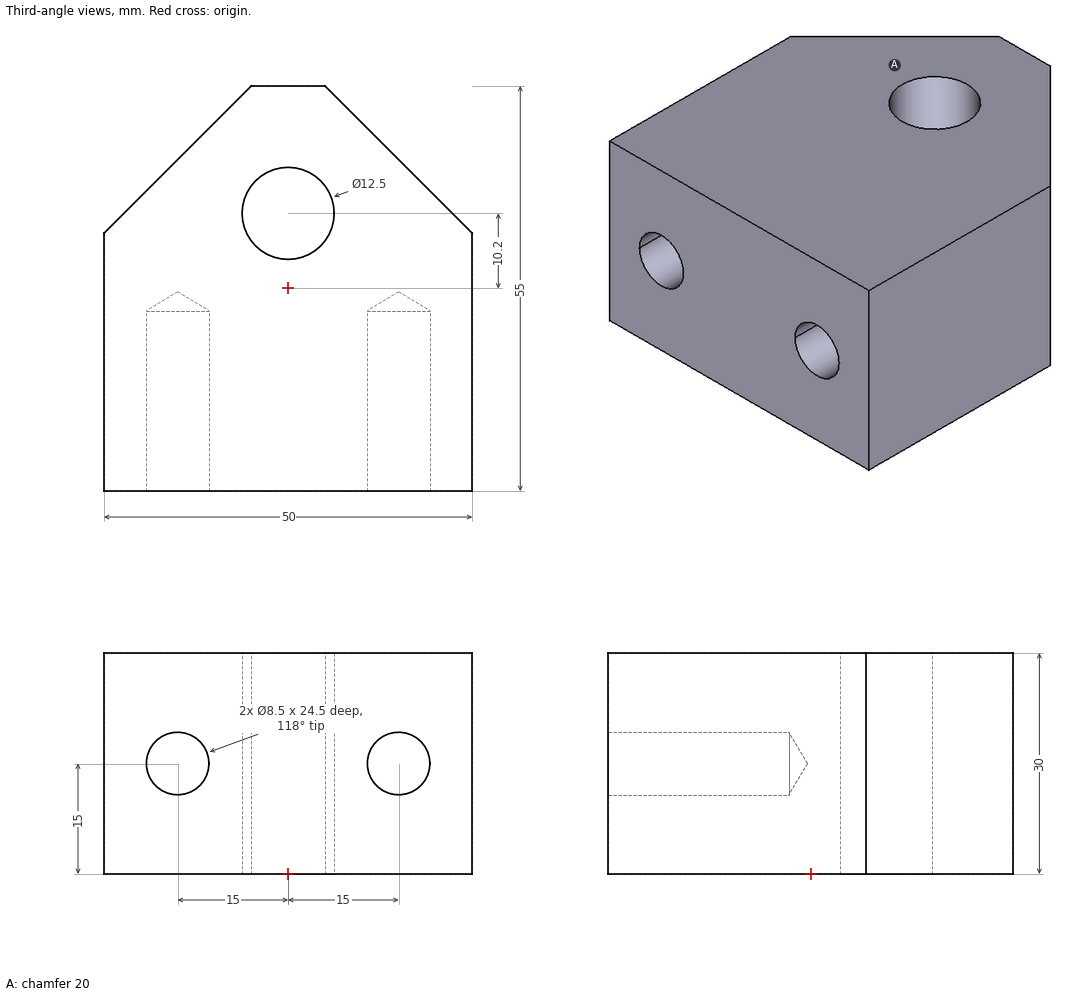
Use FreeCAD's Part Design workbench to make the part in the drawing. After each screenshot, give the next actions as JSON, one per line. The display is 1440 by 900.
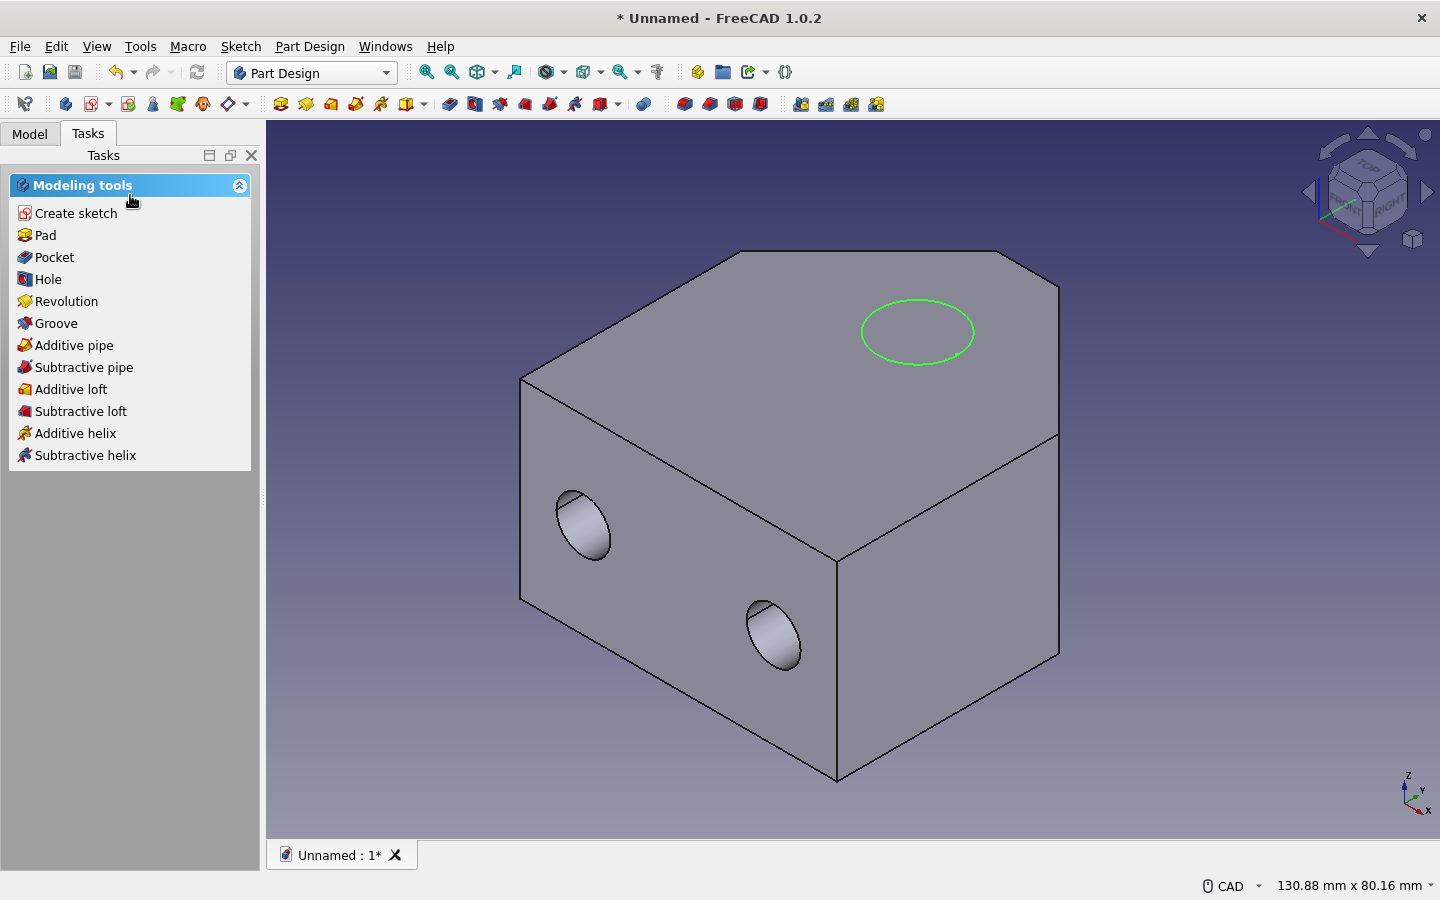
{"action": "left_click", "coordinate": [450, 104]}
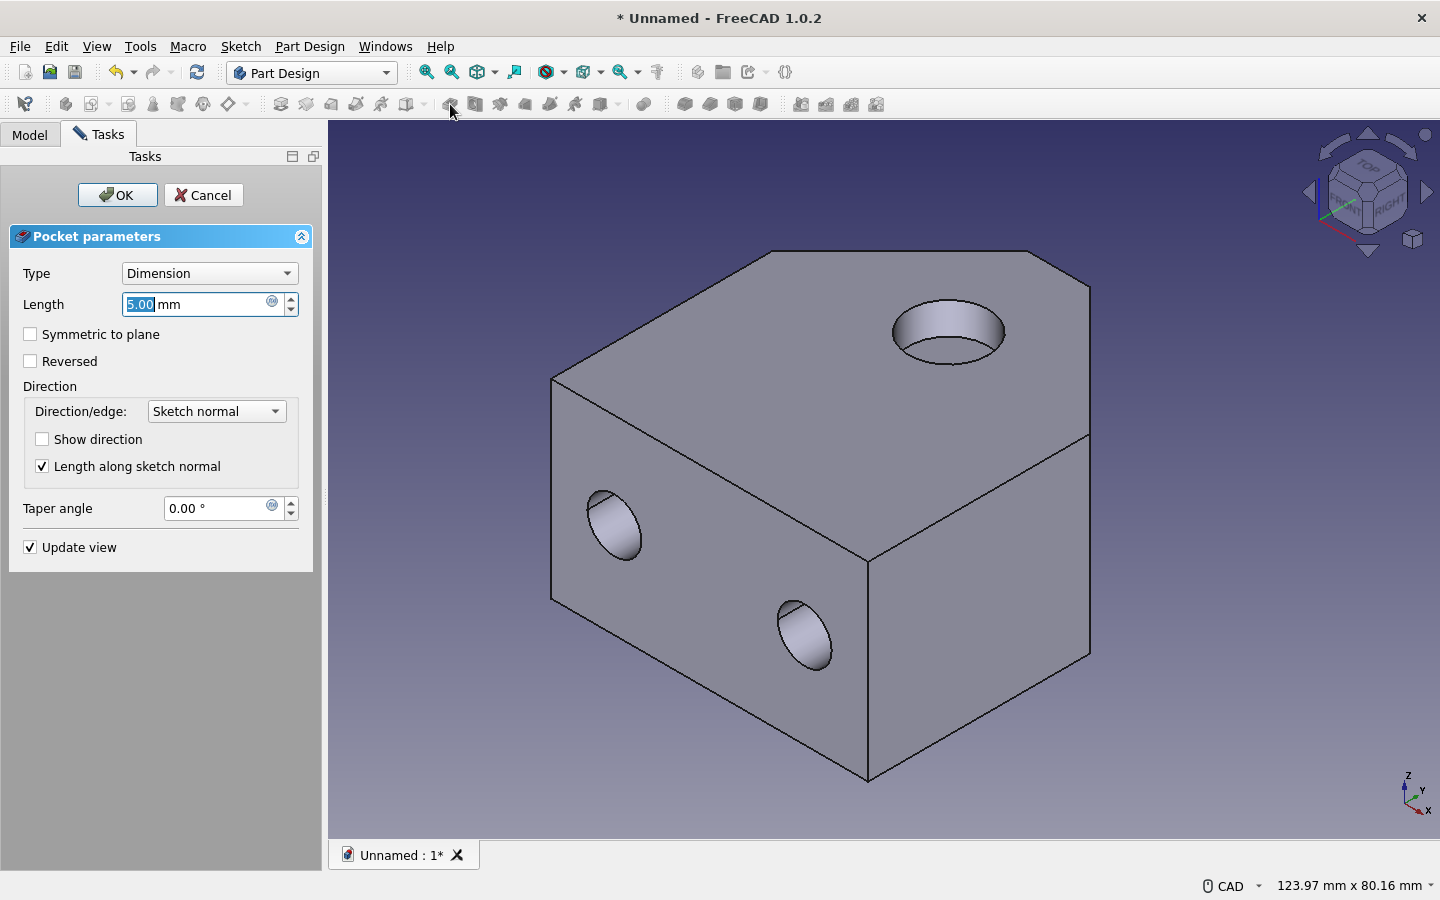
{"action": "type", "text": "30"}
{"action": "key", "text": "Tab"}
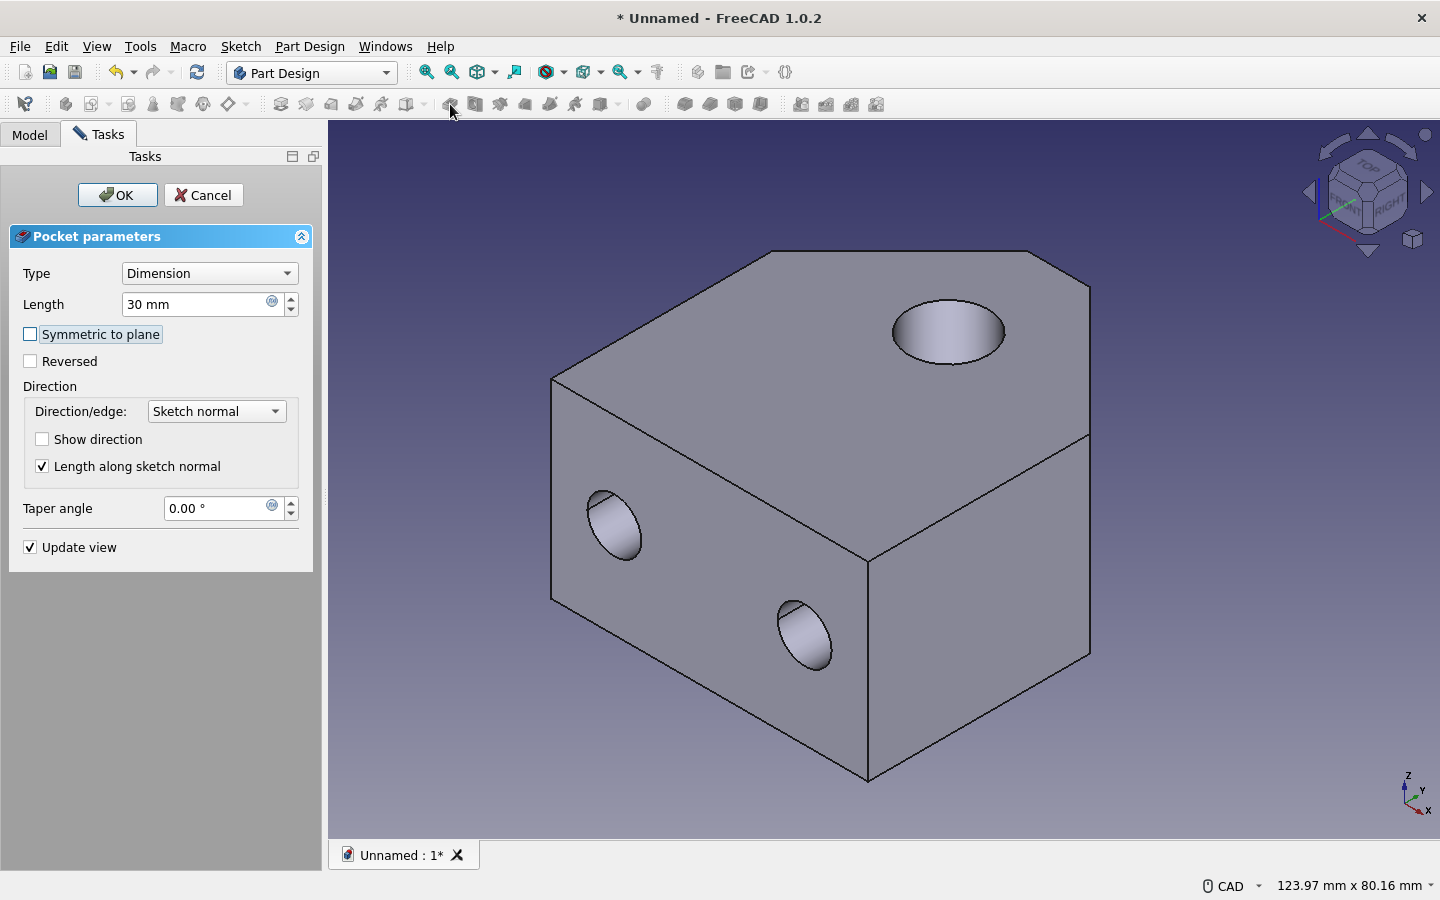
{"action": "left_click", "coordinate": [118, 195]}